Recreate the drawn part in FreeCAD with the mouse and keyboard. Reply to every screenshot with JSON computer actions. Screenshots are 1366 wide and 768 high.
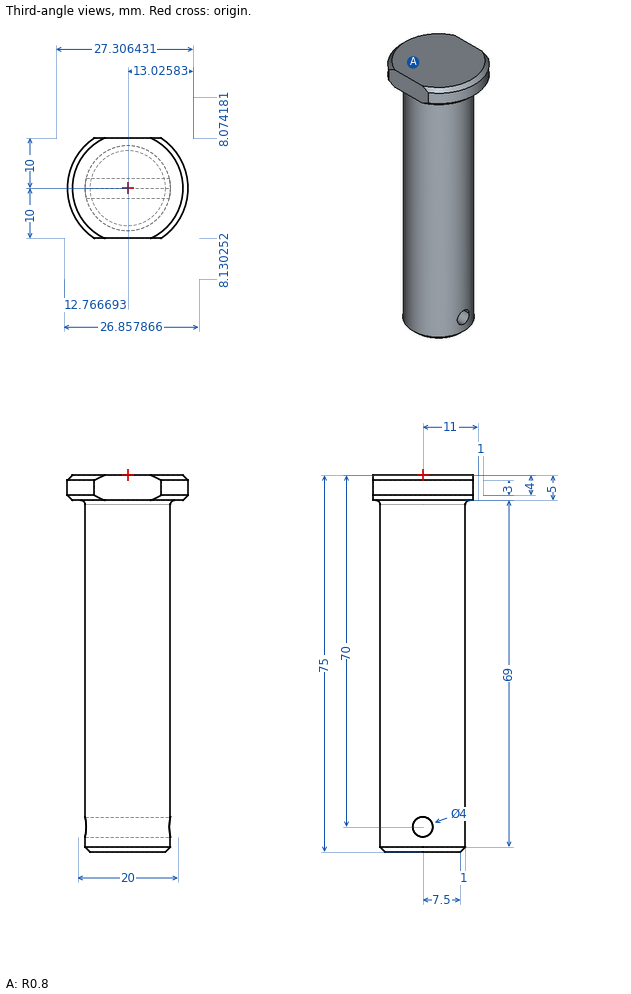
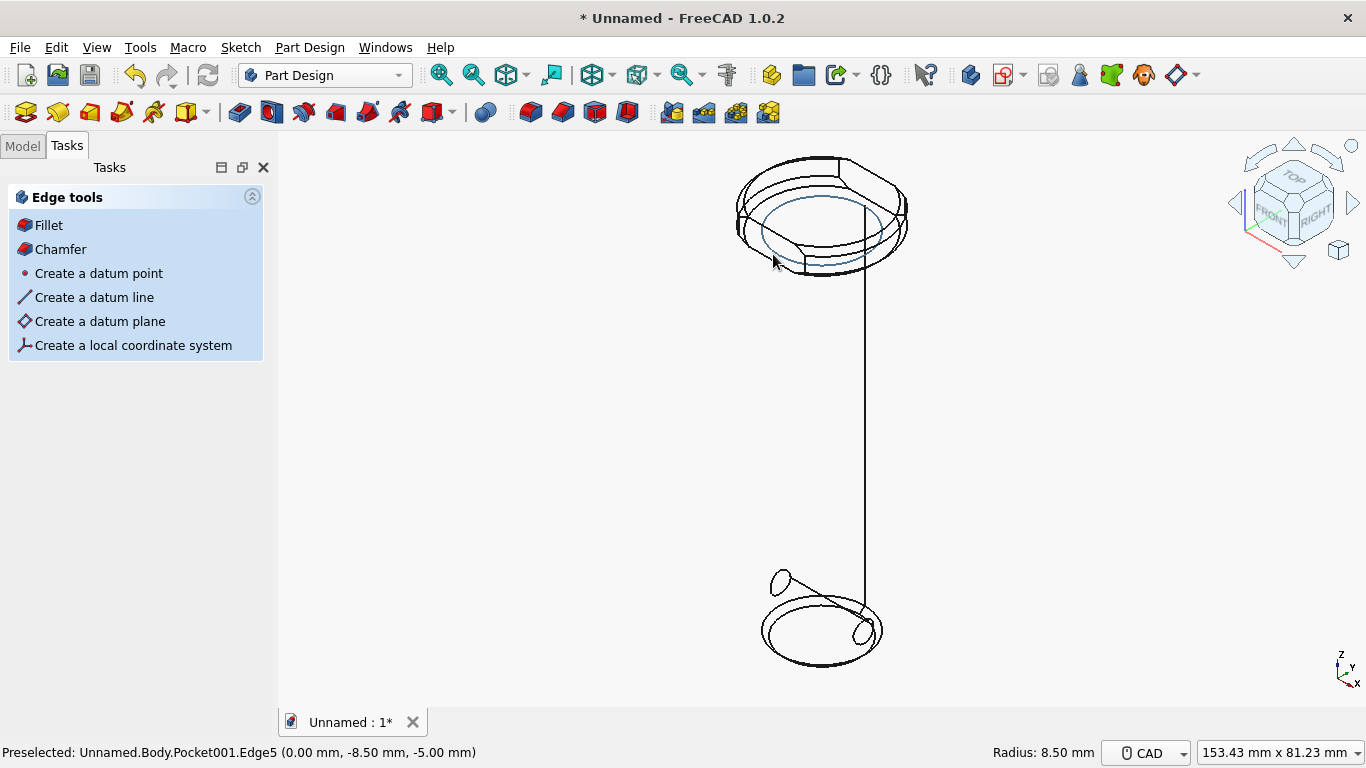
{"action": "key", "text": "v 1"}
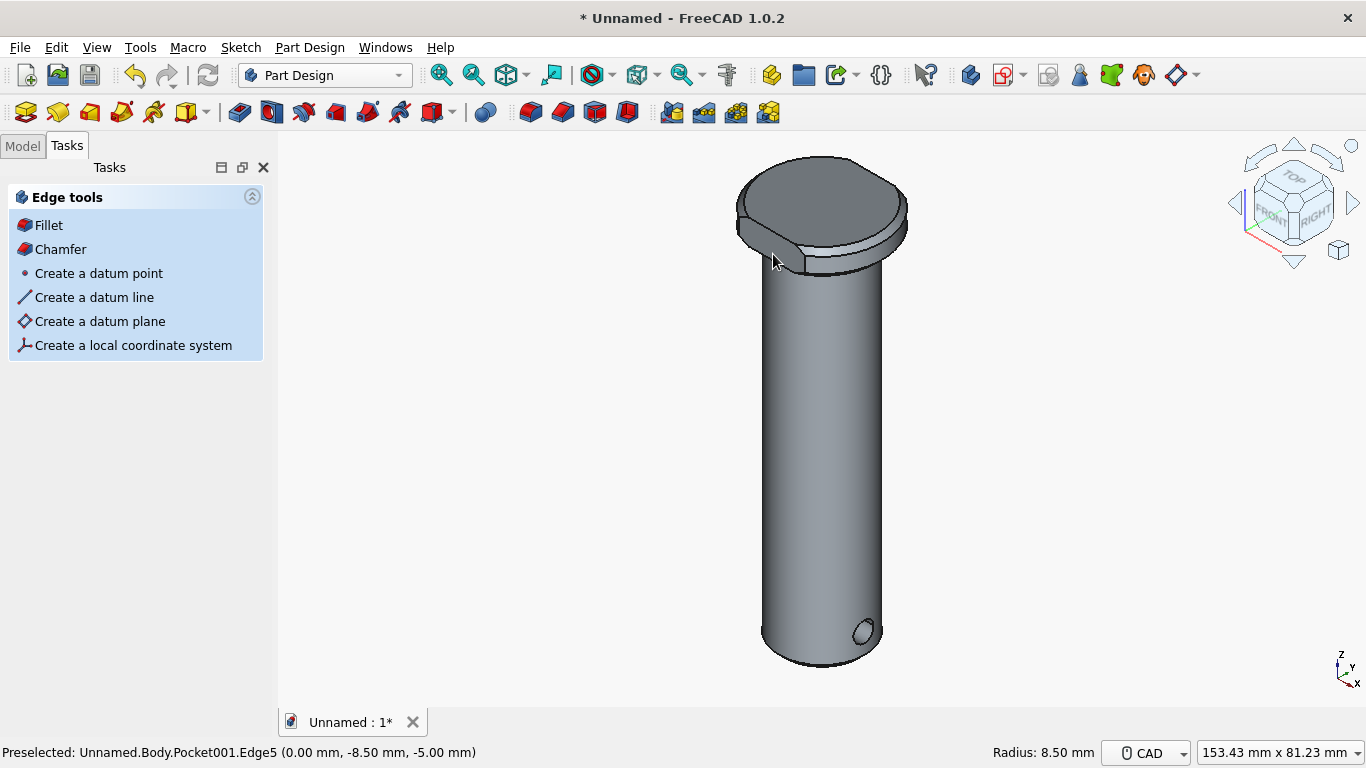
{"action": "left_click", "coordinate": [532, 112]}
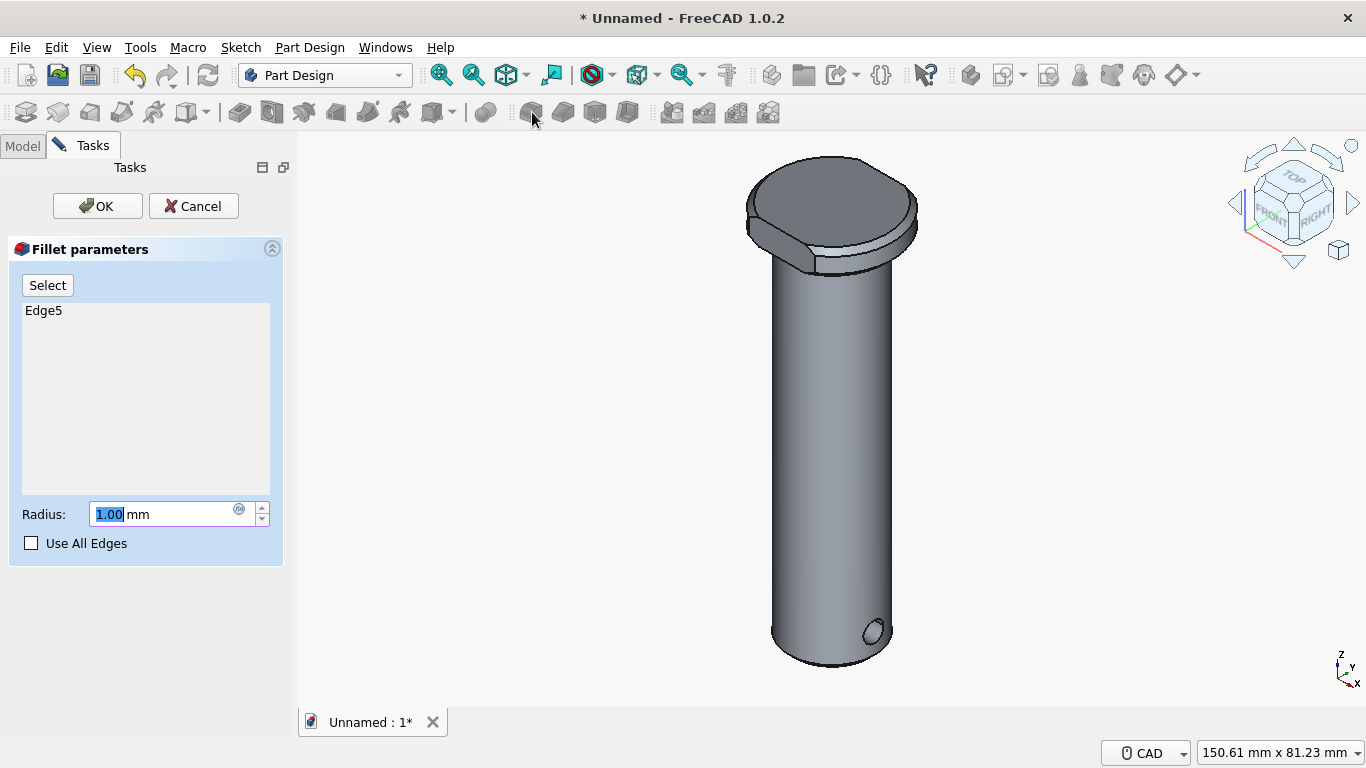
{"action": "type", "text": "0.8"}
{"action": "key", "text": "Tab"}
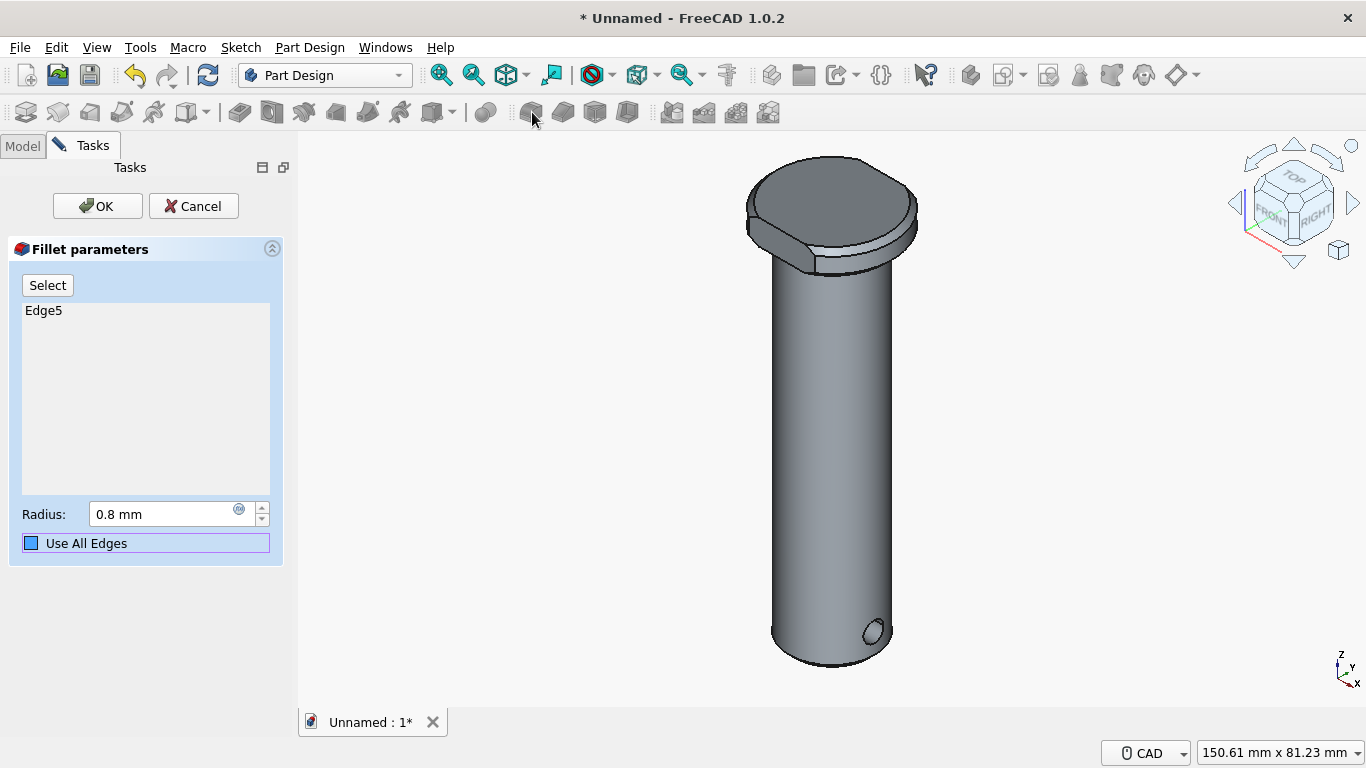
{"action": "left_click", "coordinate": [98, 206]}